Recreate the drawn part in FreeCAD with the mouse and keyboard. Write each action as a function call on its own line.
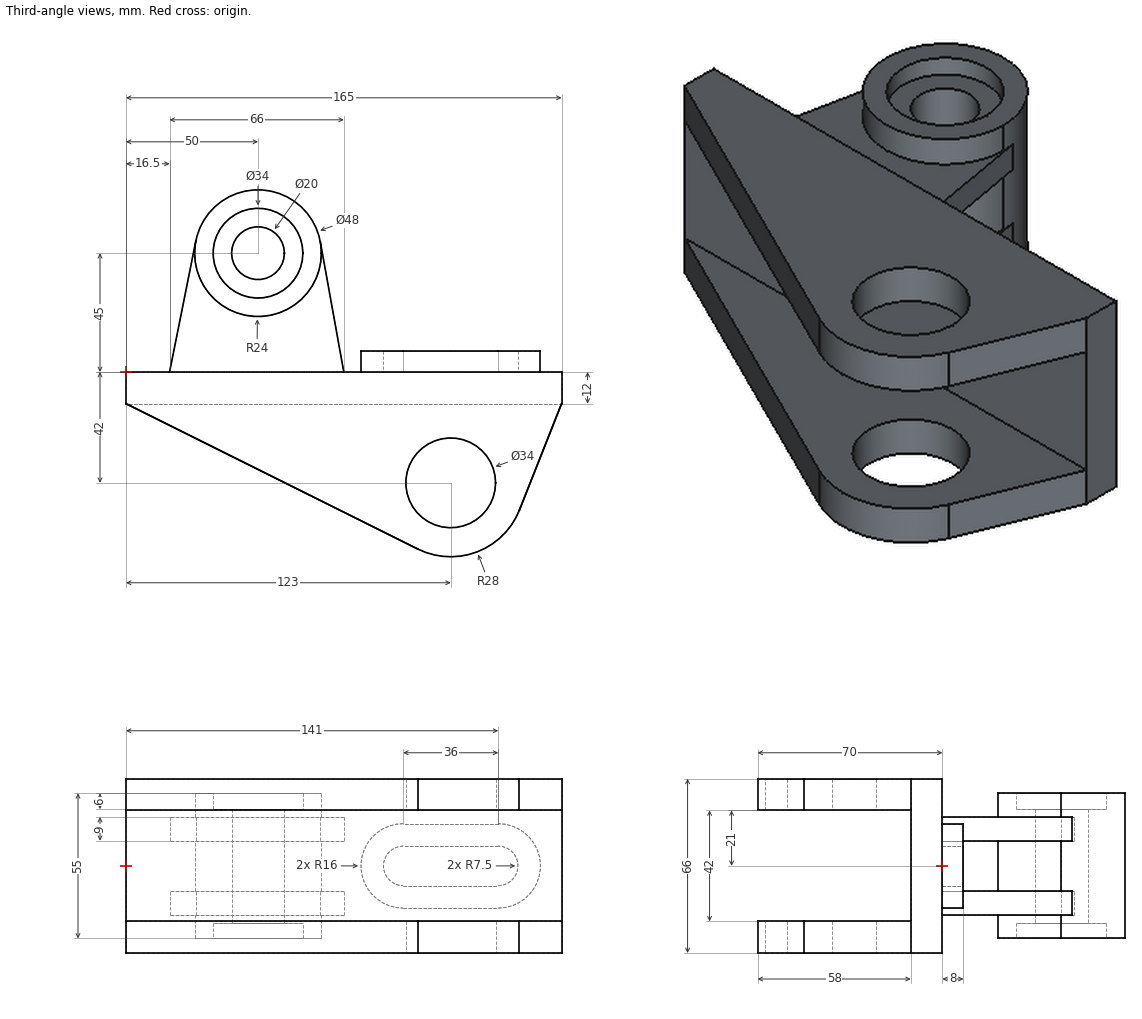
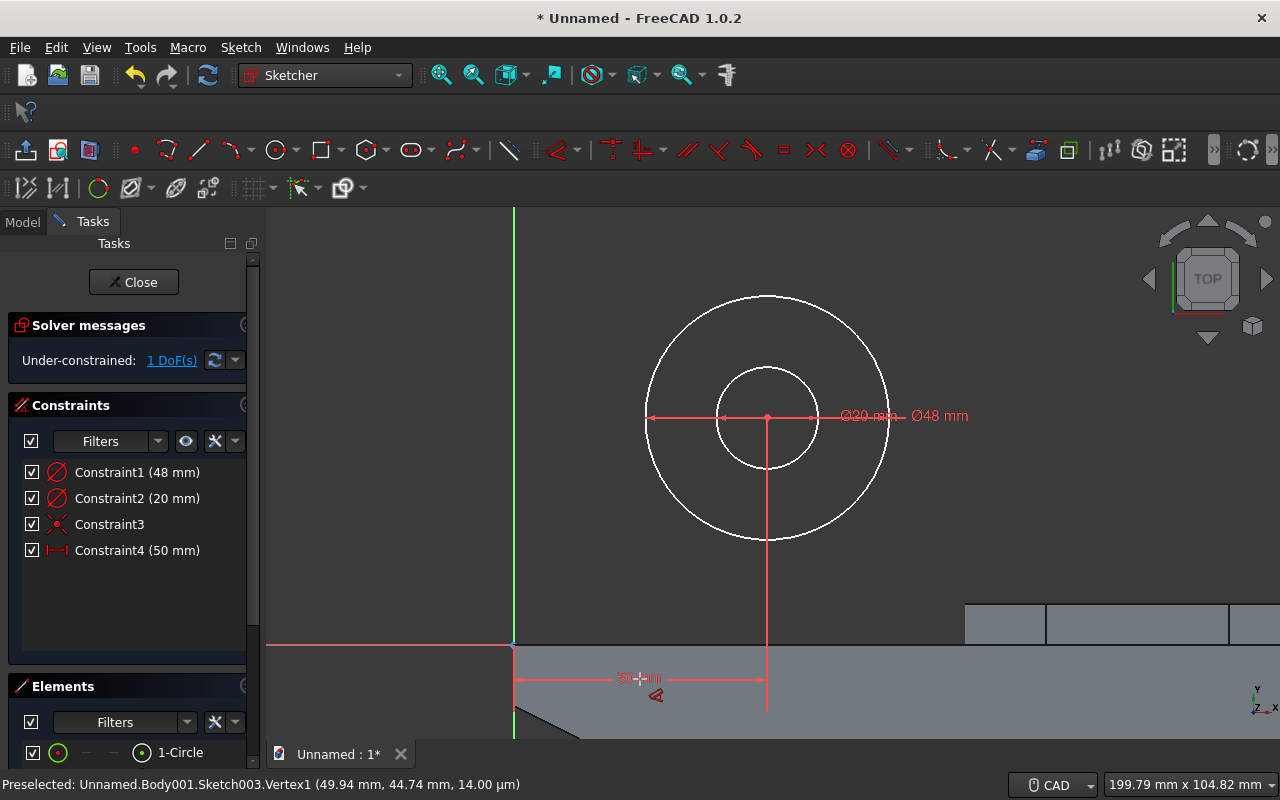
click(767, 418)
click(480, 532)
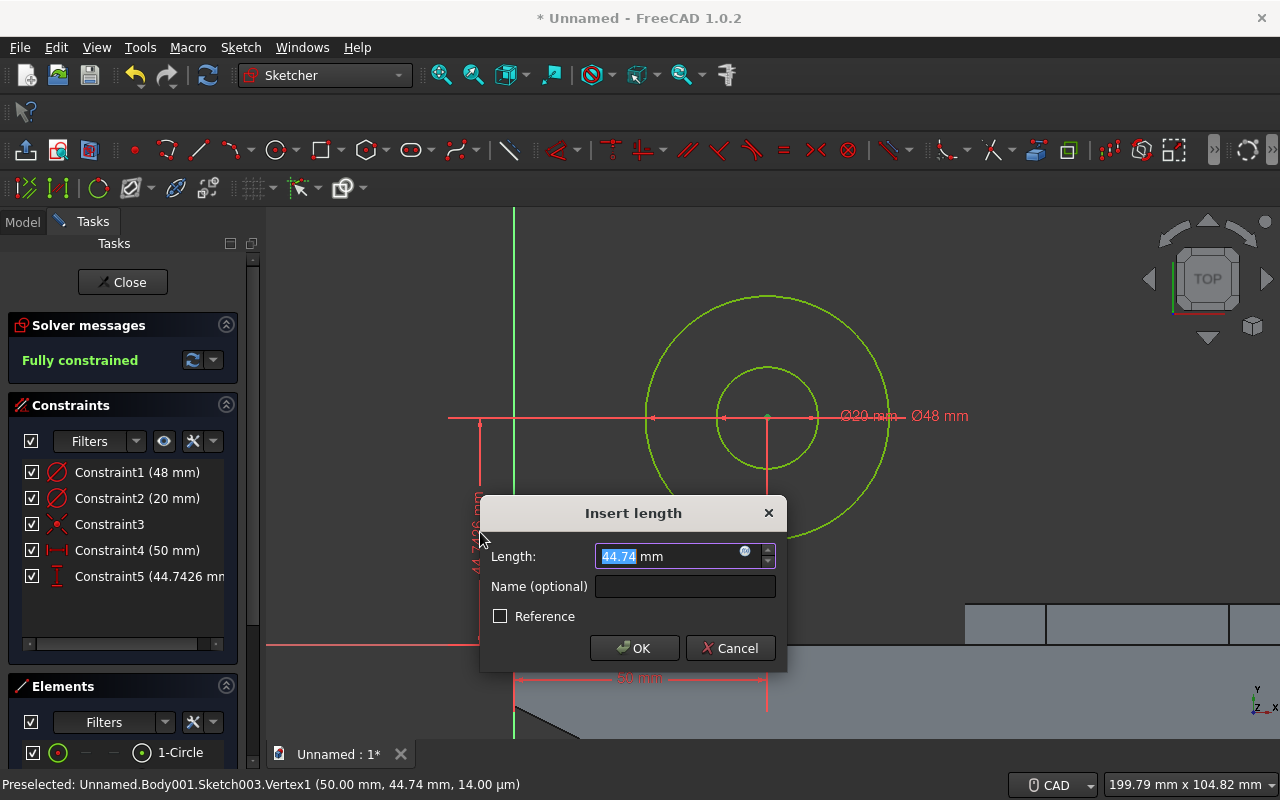
text(45)
key(Return)
key(Escape)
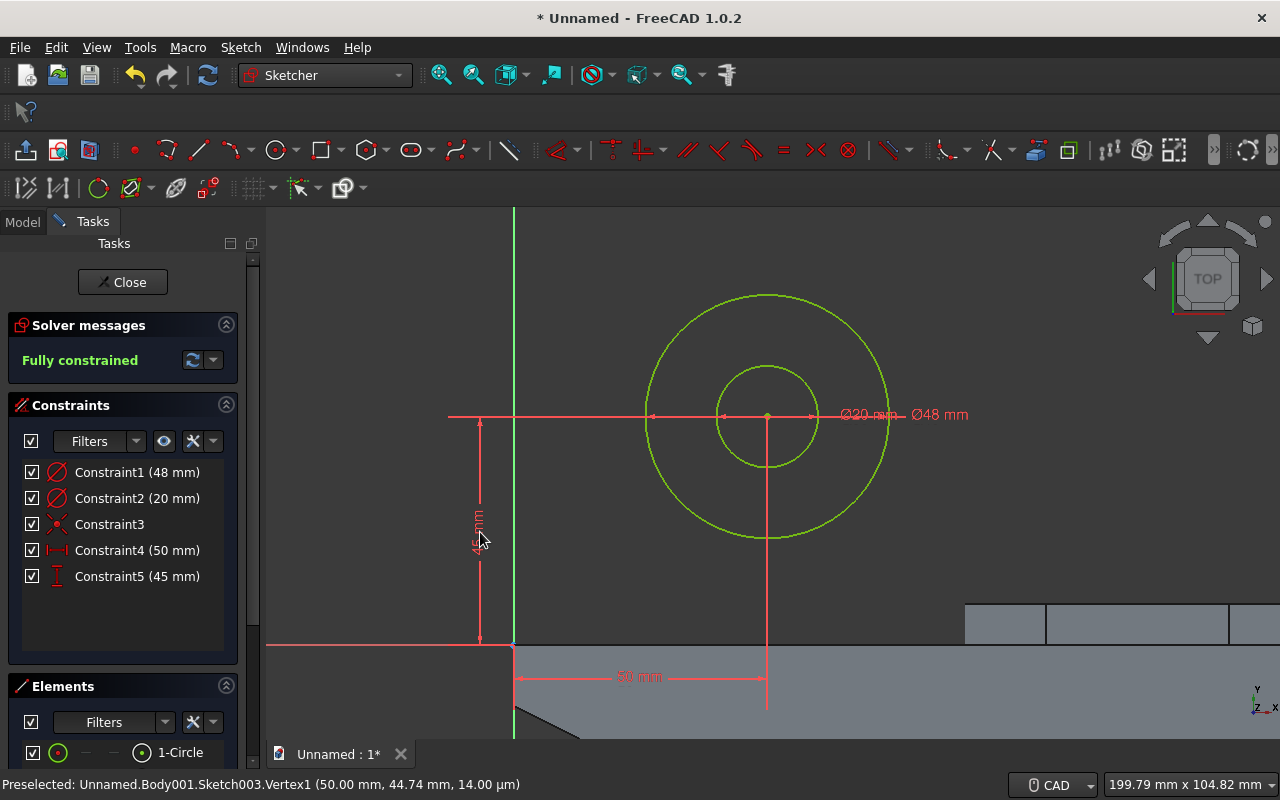
click(123, 282)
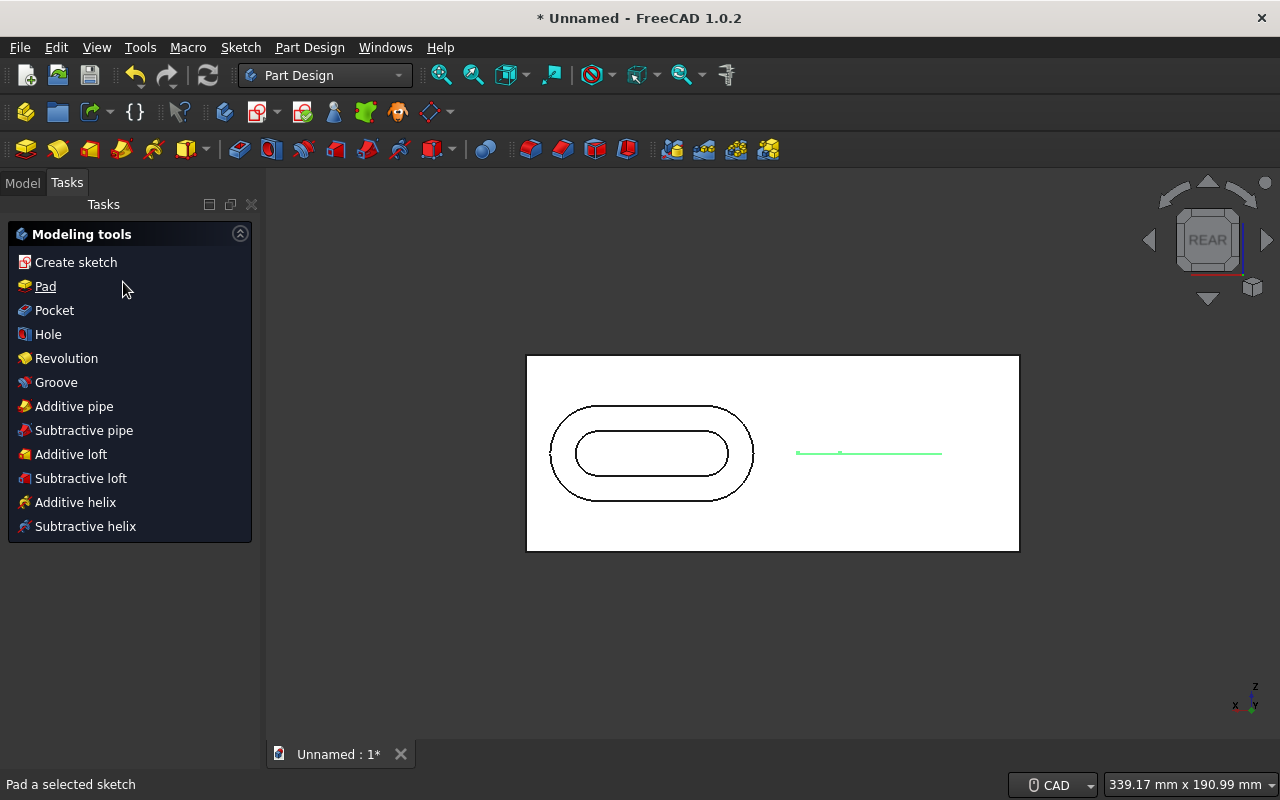
click(26, 150)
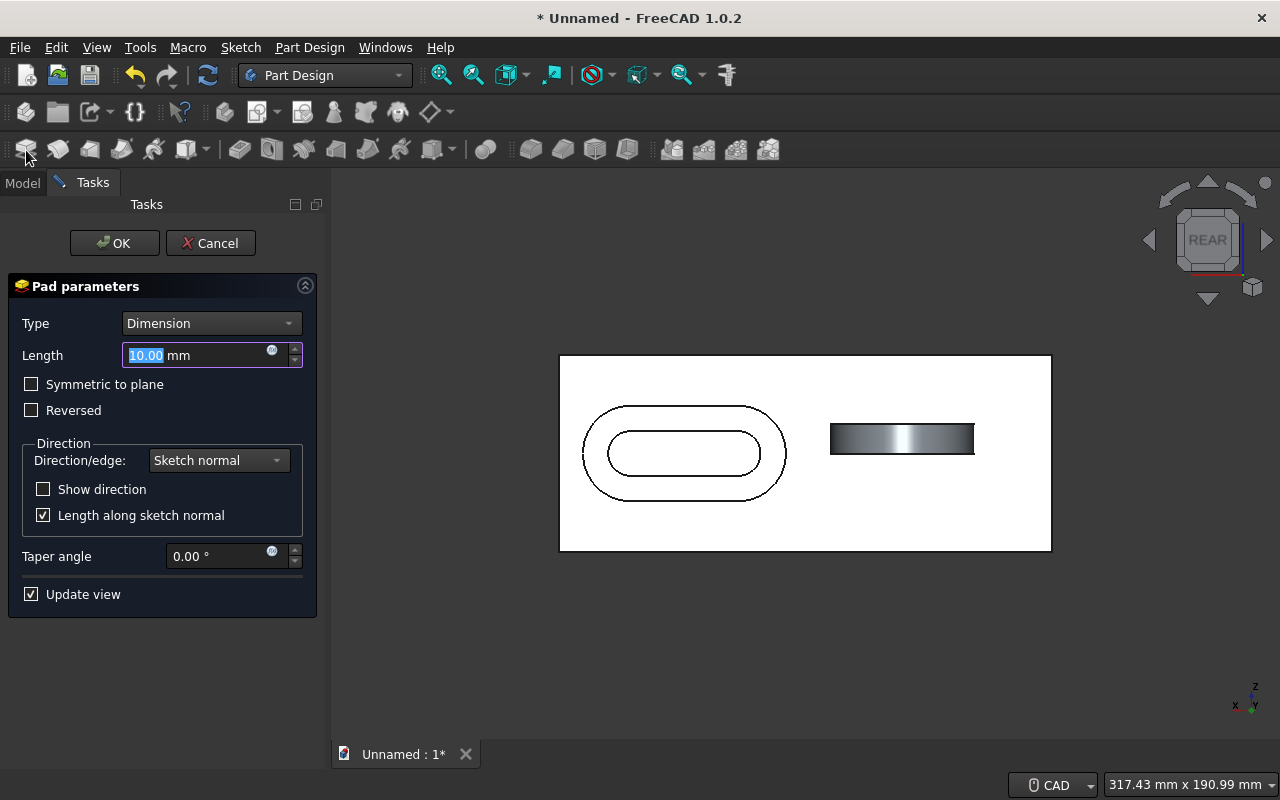
text(55)
key(Tab)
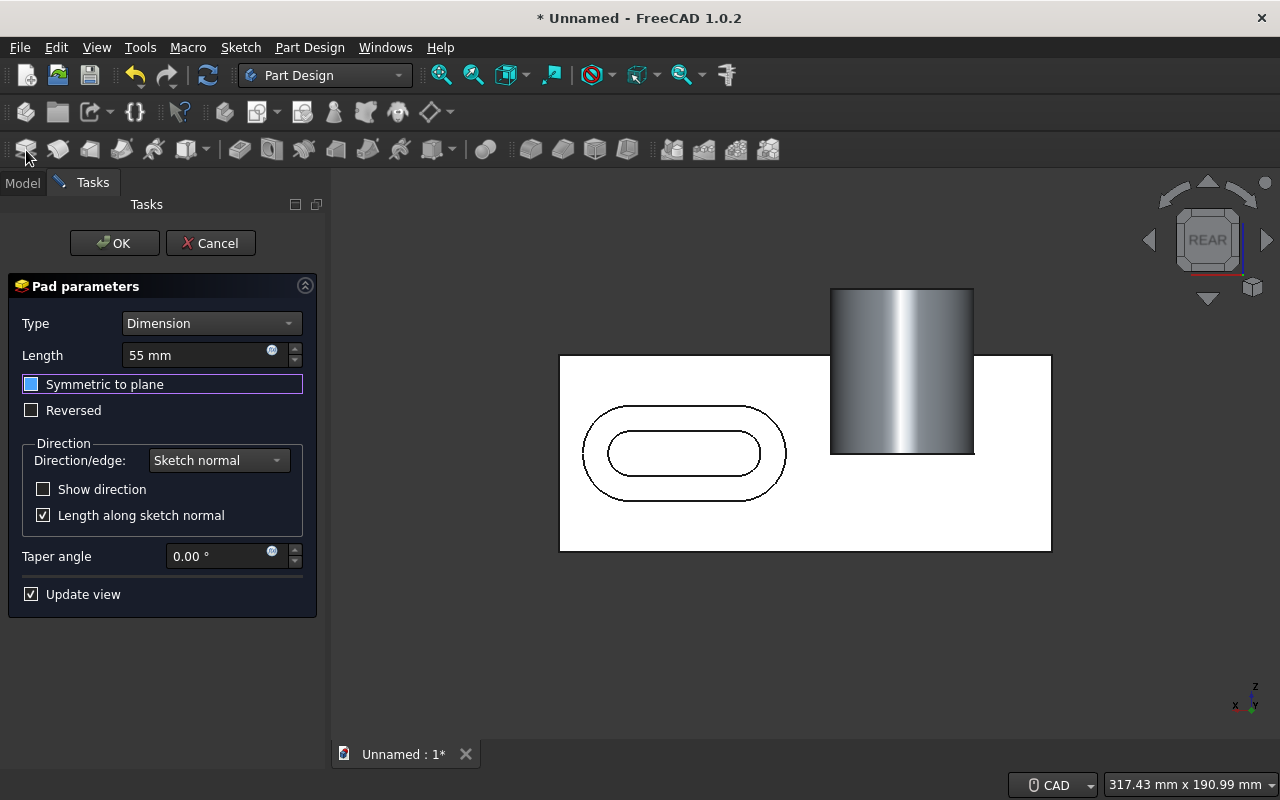
click(30, 384)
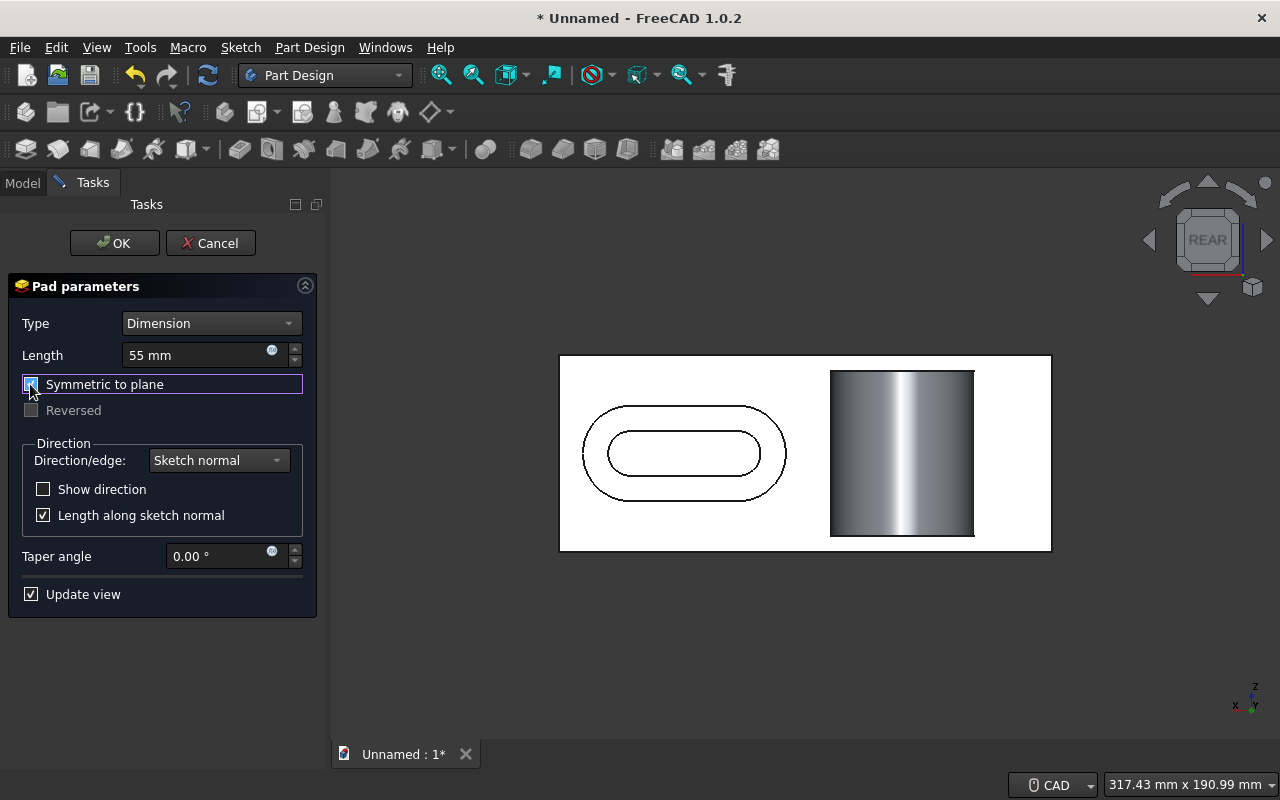
click(115, 243)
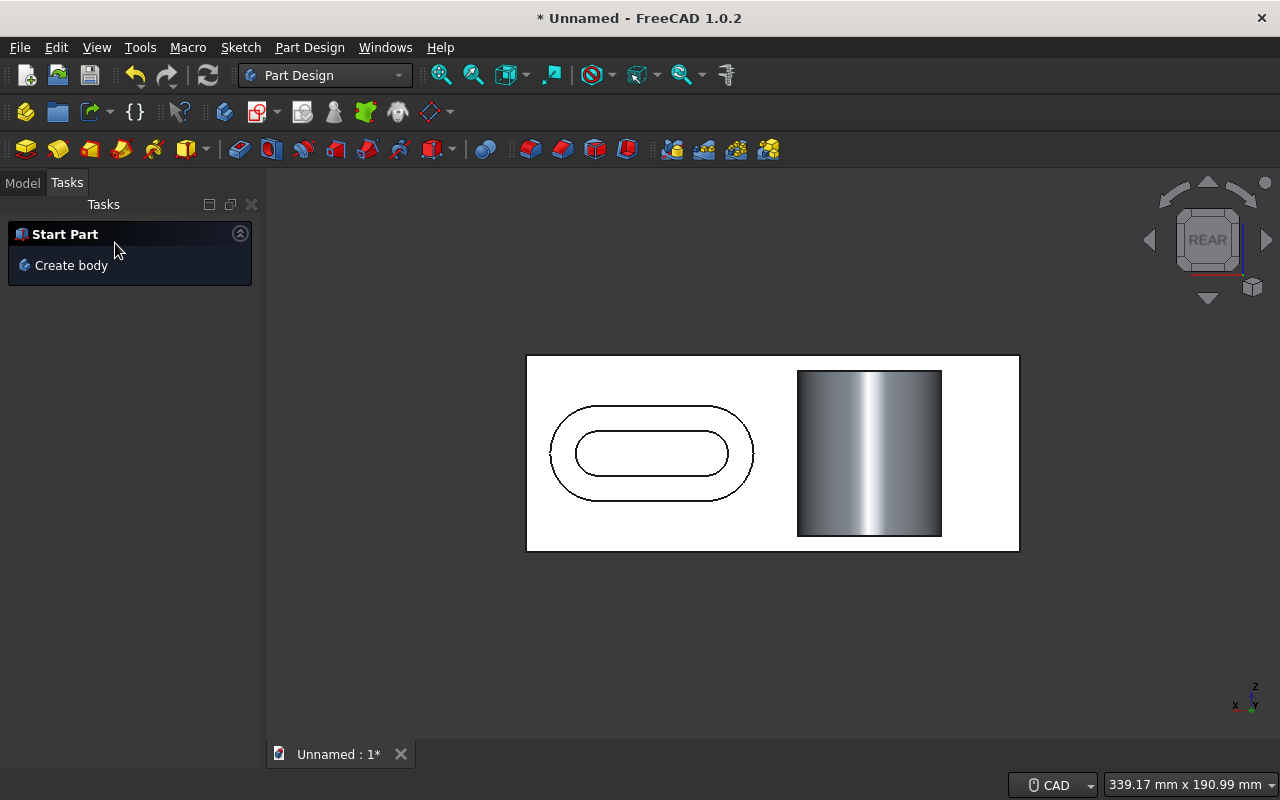
click(442, 76)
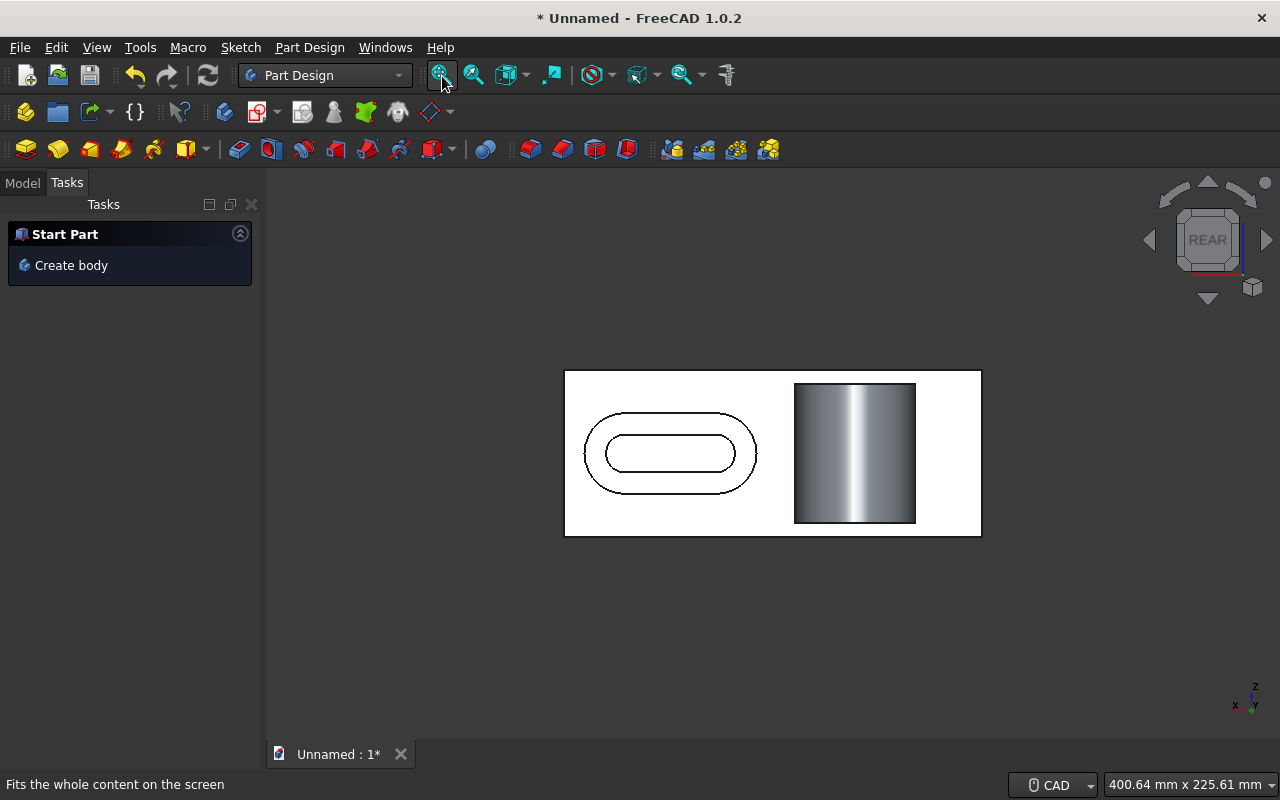
click(23, 182)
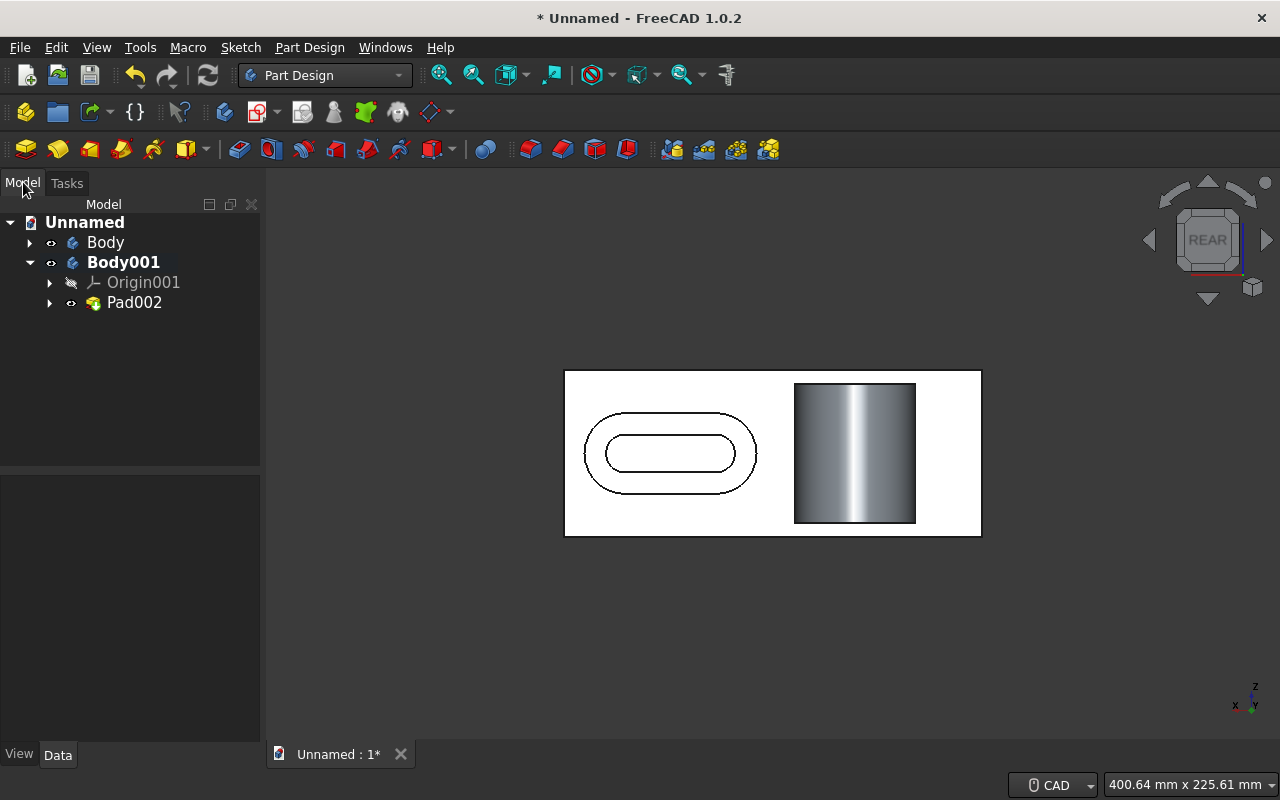
double_click(96, 243)